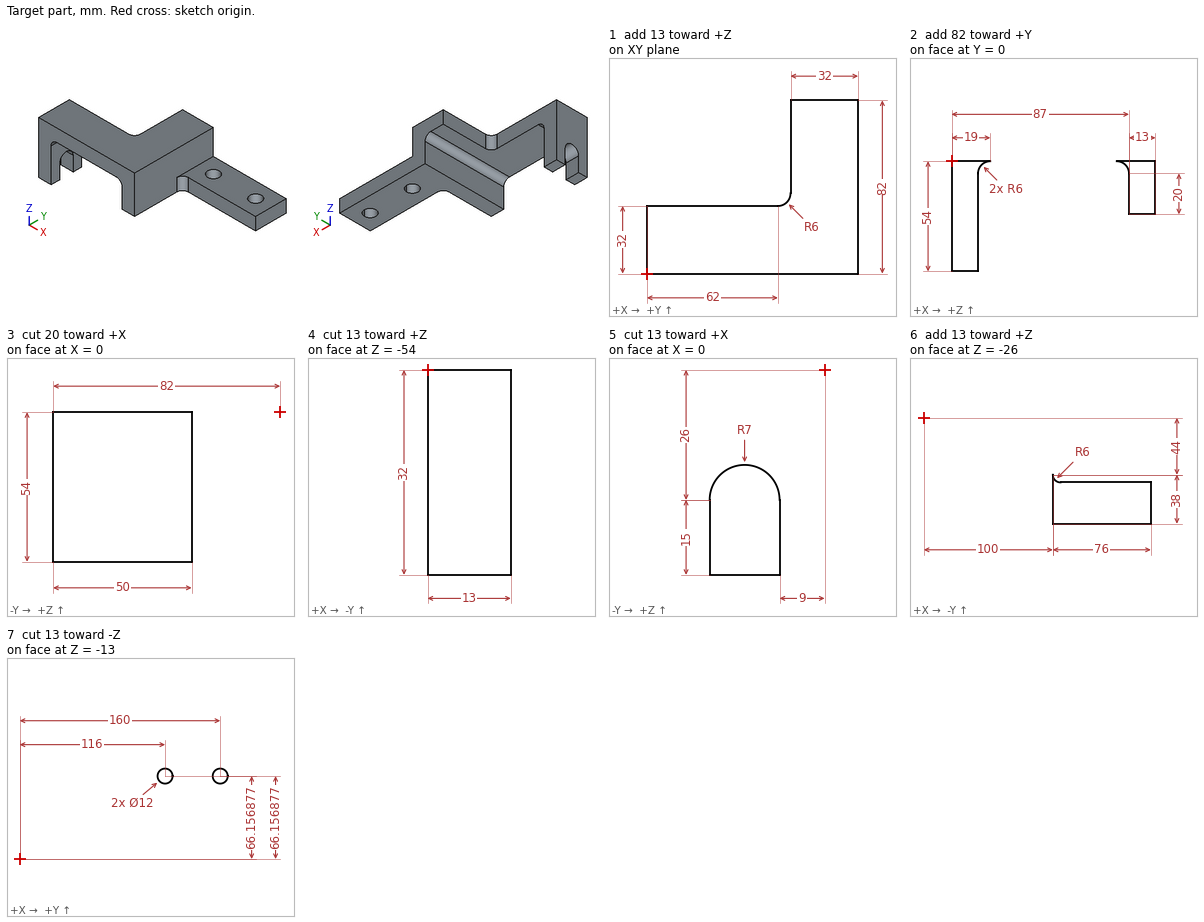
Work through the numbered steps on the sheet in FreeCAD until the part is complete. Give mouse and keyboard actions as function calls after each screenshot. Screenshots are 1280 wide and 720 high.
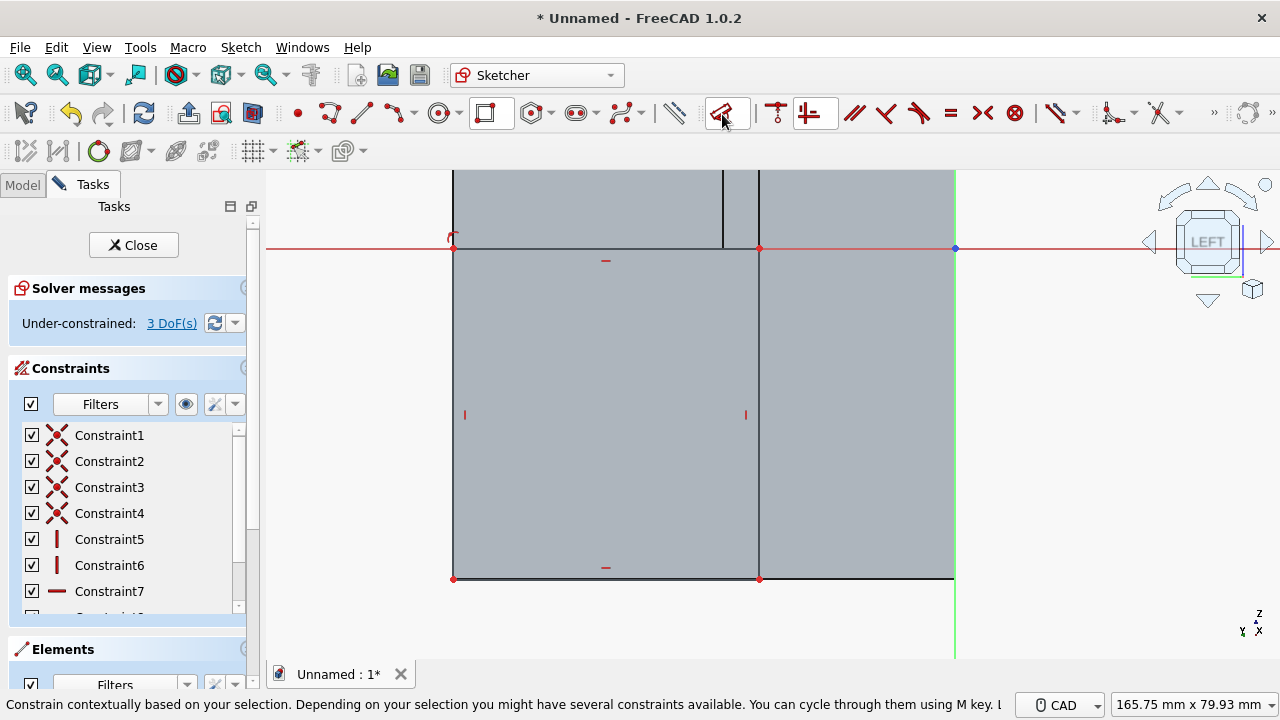
click(453, 348)
click(419, 414)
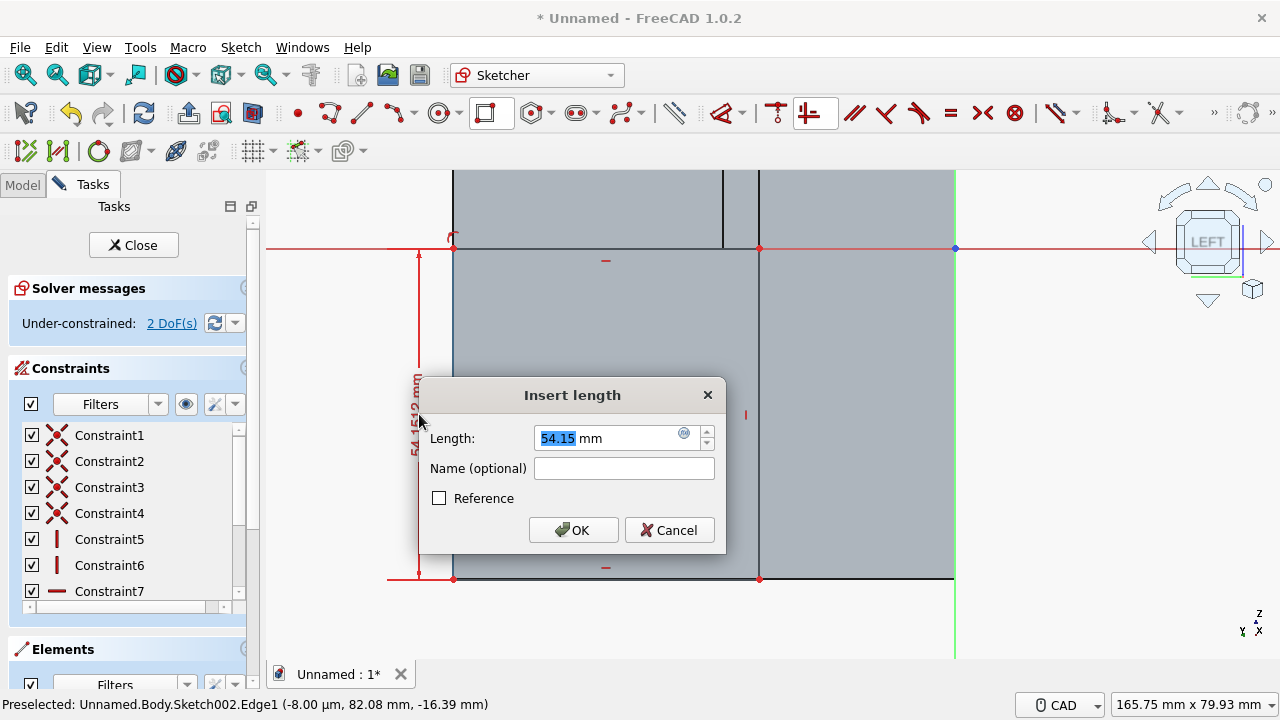
text(54)
key(Return)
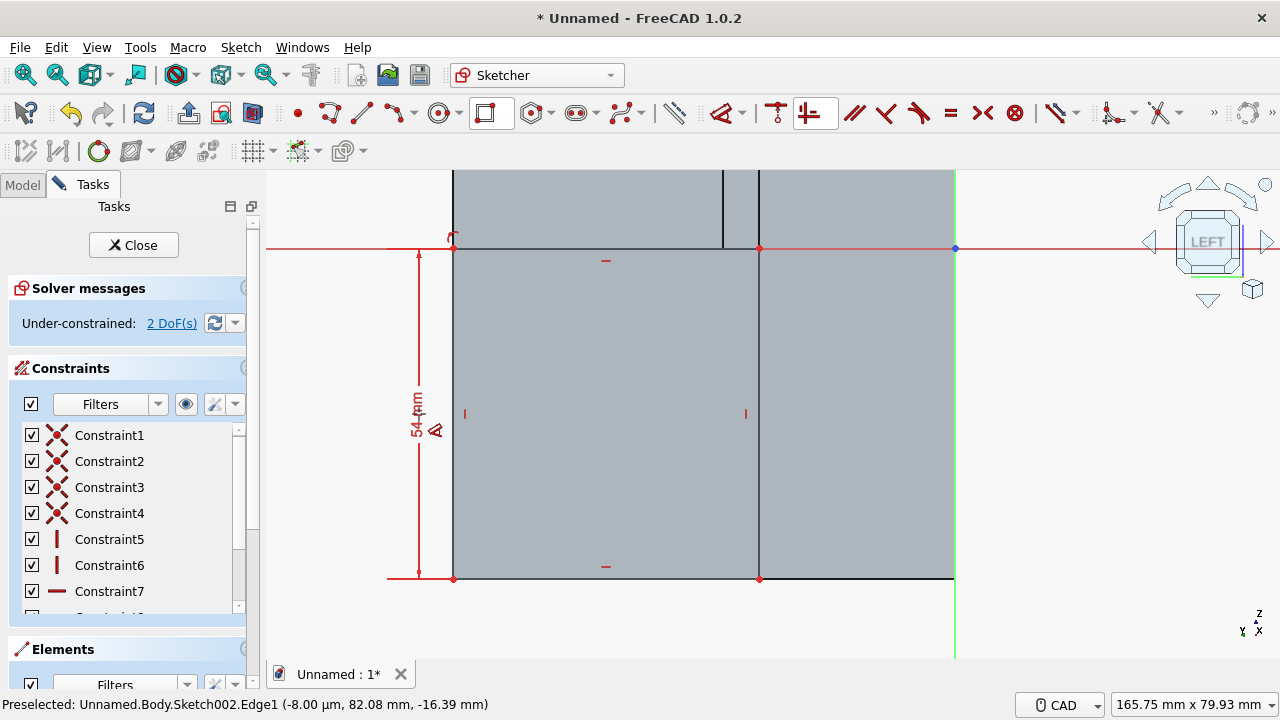
click(545, 579)
click(606, 613)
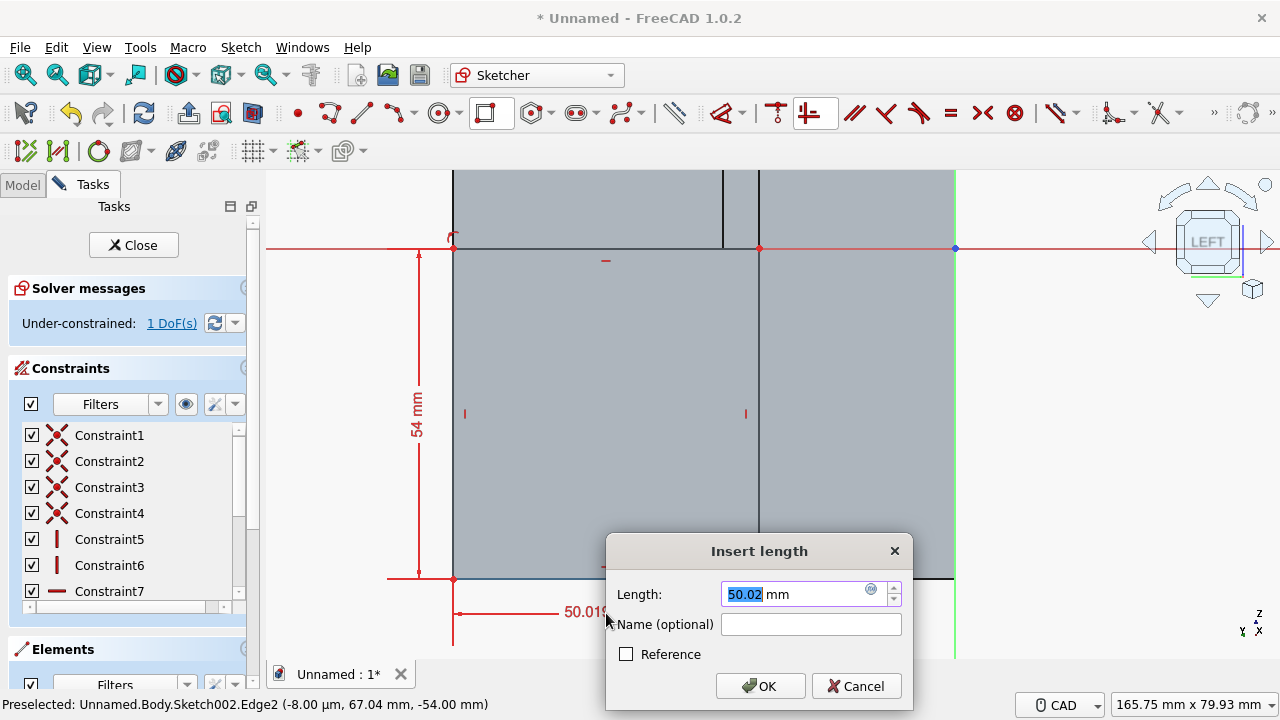
text(50)
key(Return)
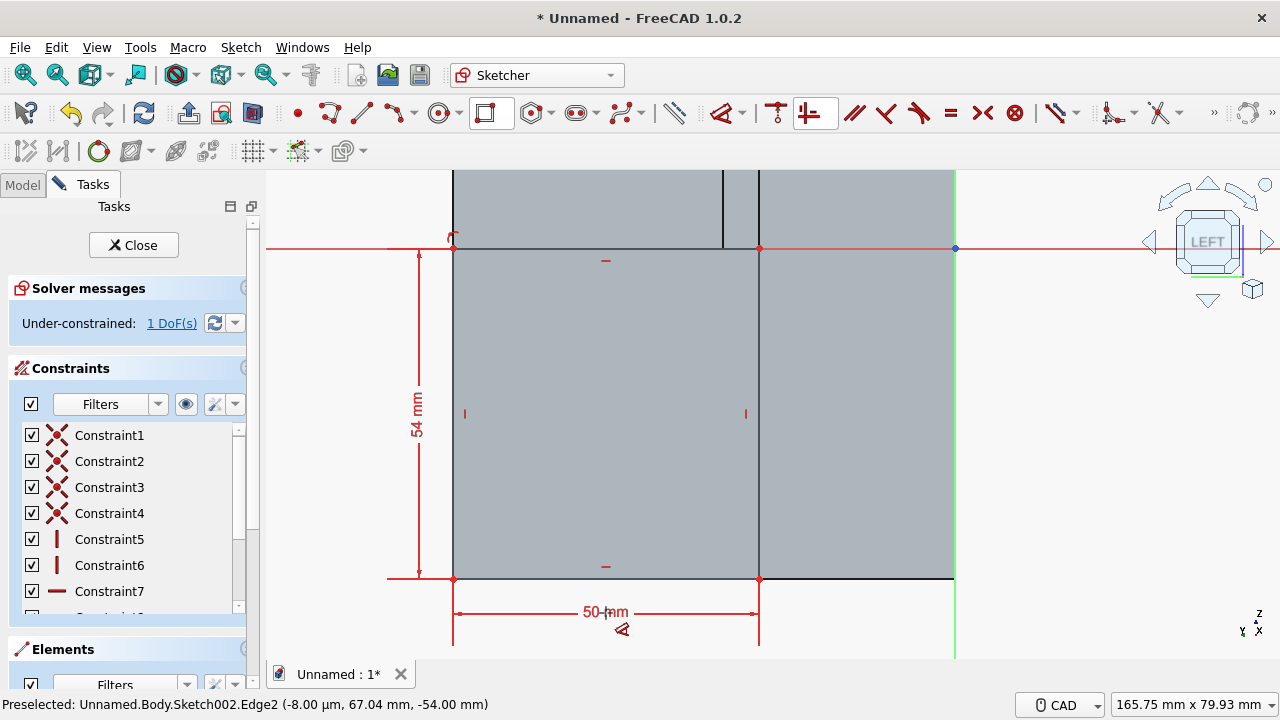
click(453, 249)
click(704, 215)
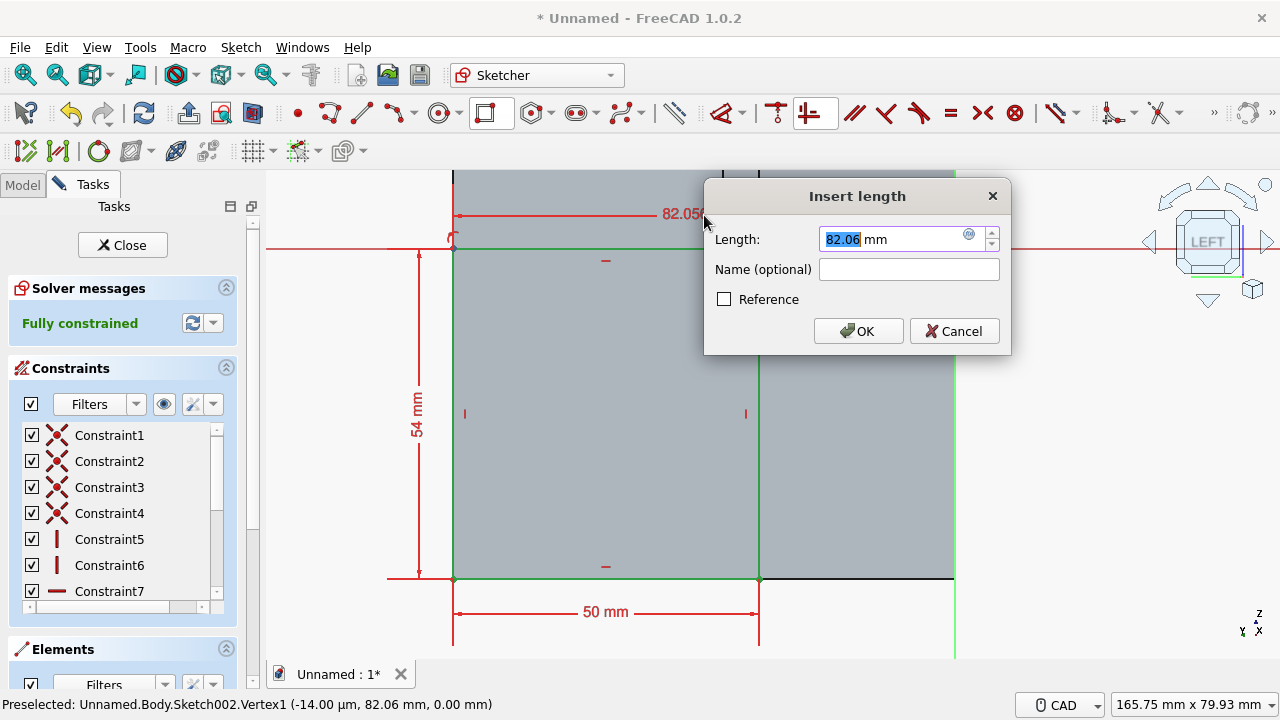
text(82)
key(Return)
key(Escape)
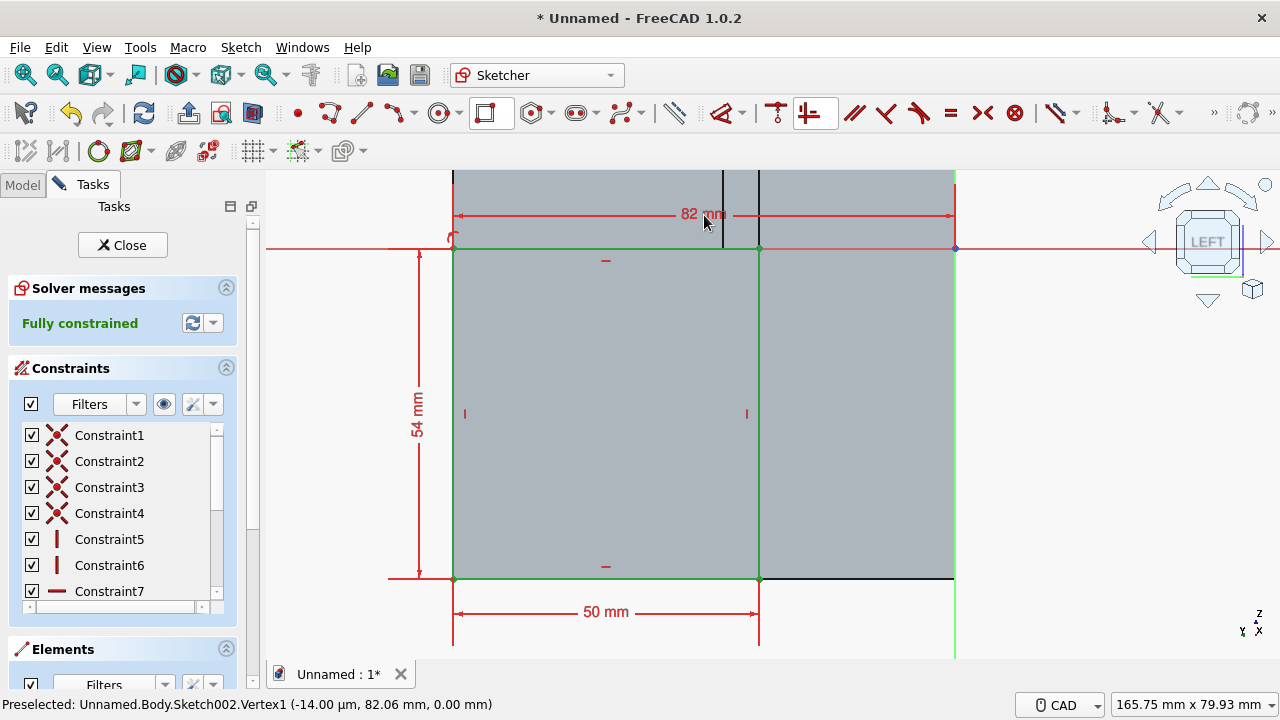
click(123, 245)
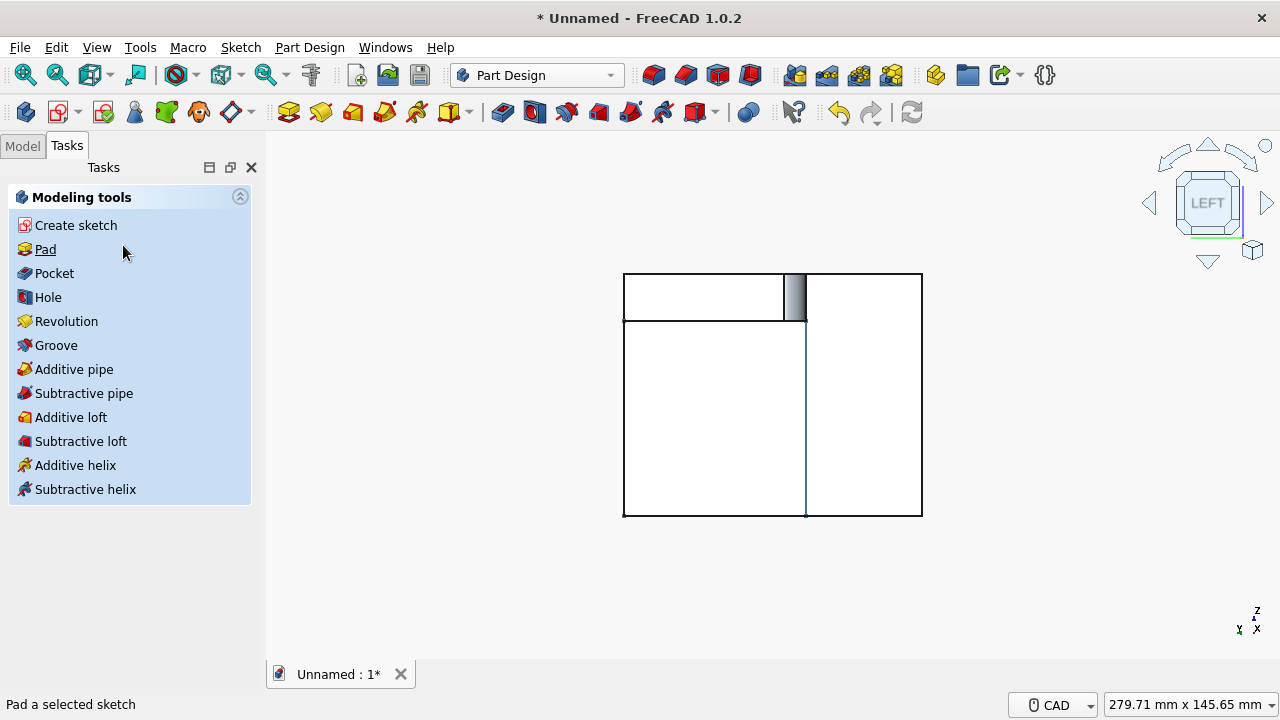
click(504, 112)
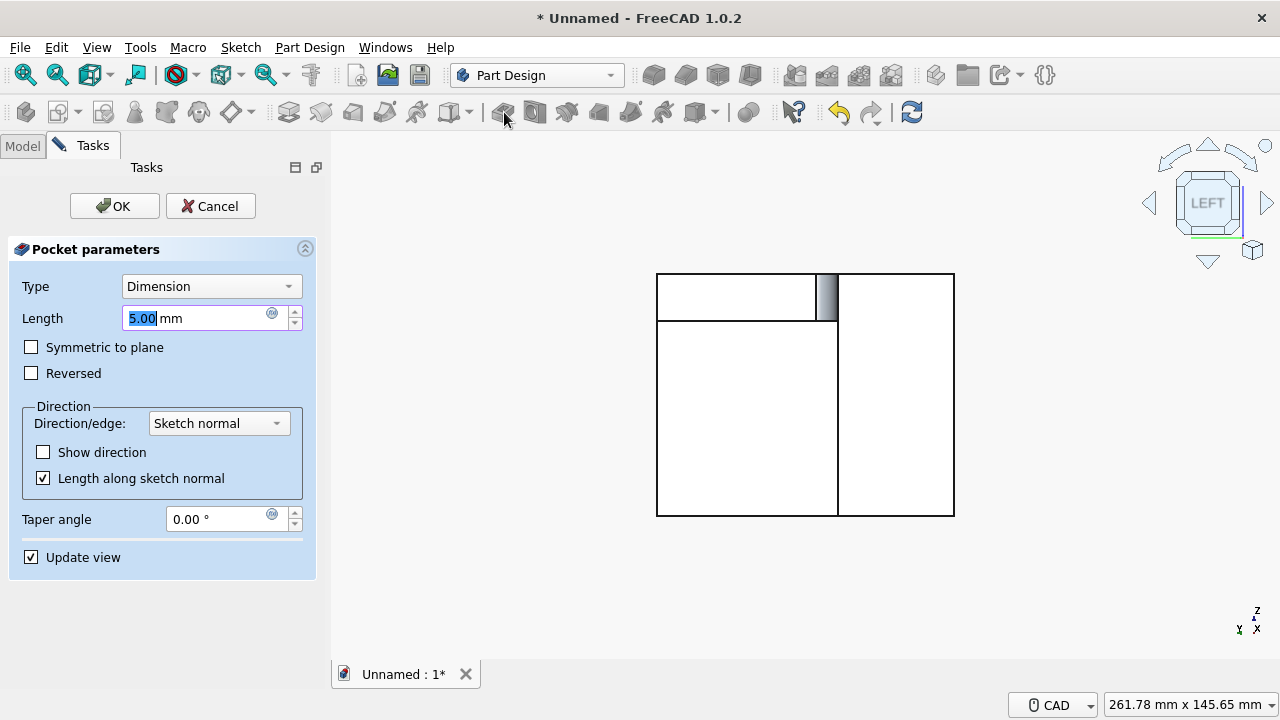
text(20)
key(Tab)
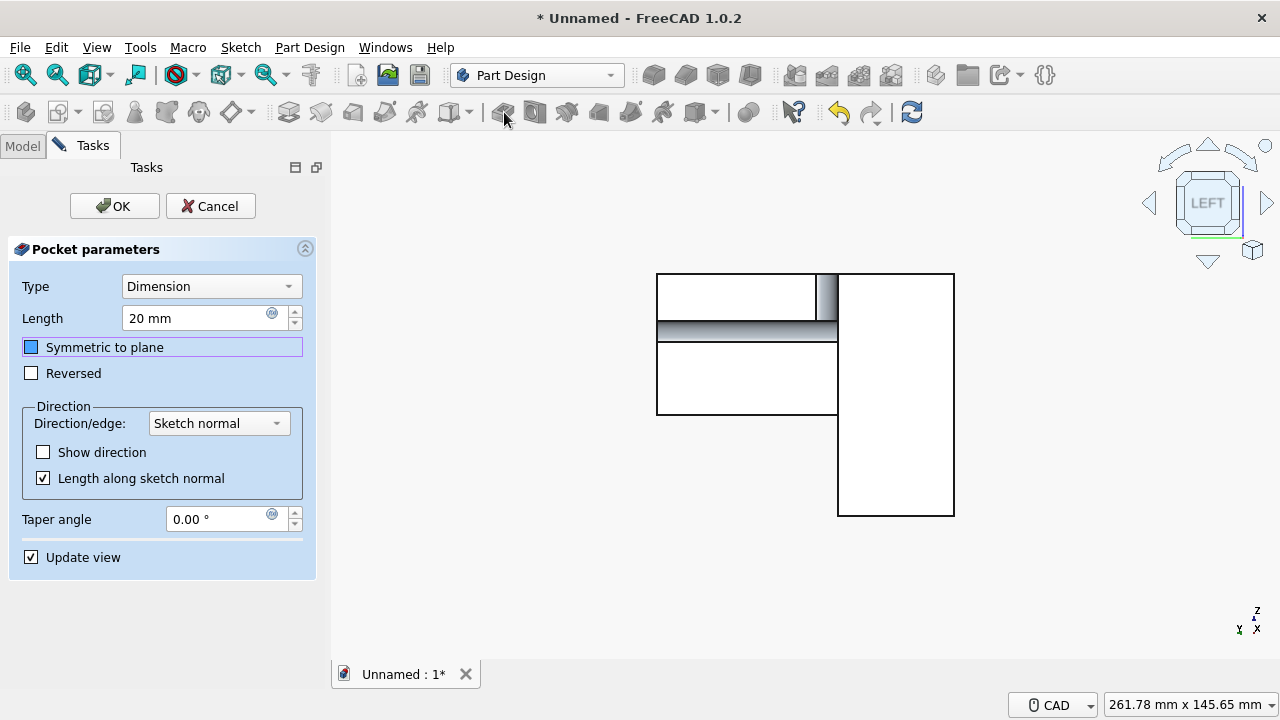
click(115, 206)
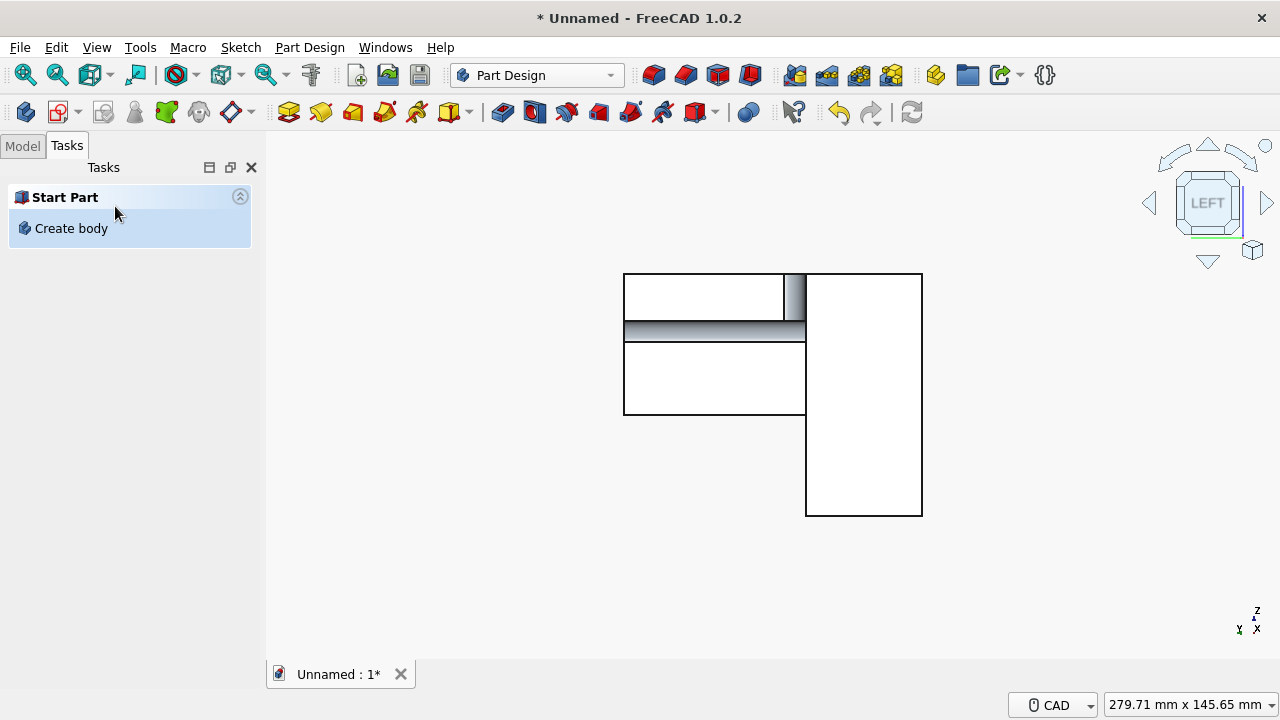
key(5)